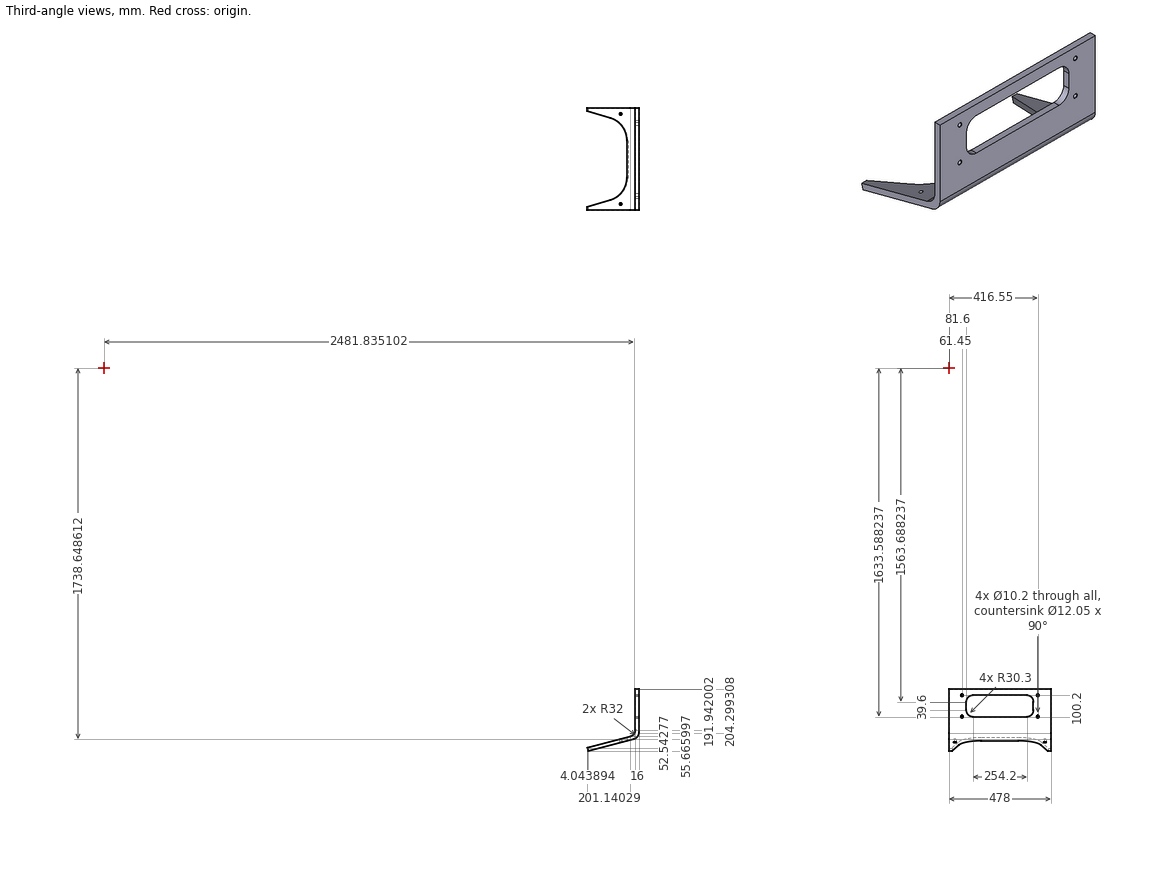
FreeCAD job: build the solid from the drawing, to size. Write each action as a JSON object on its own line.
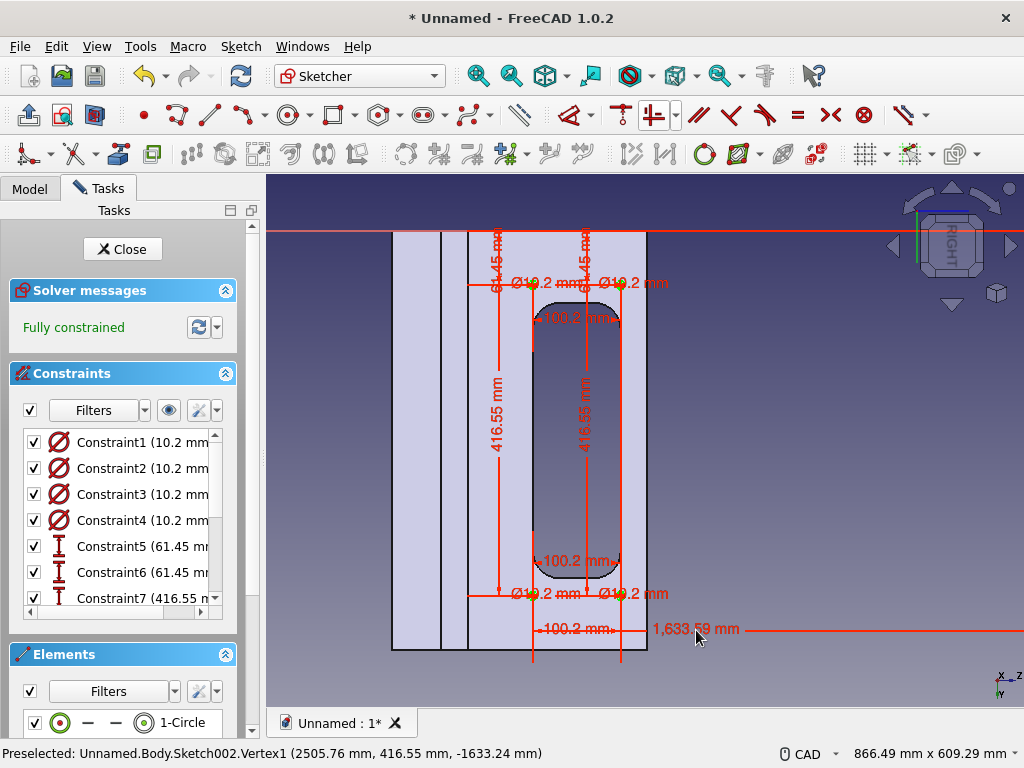
{"action": "left_click", "coordinate": [123, 249]}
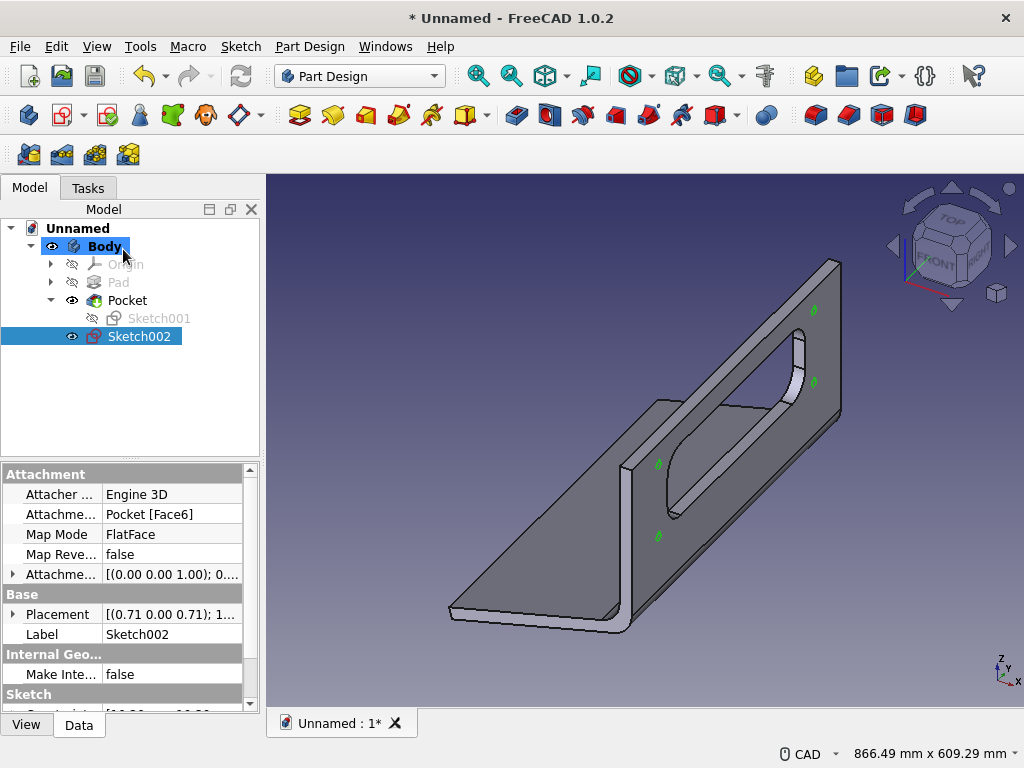
{"action": "left_click", "coordinate": [550, 116]}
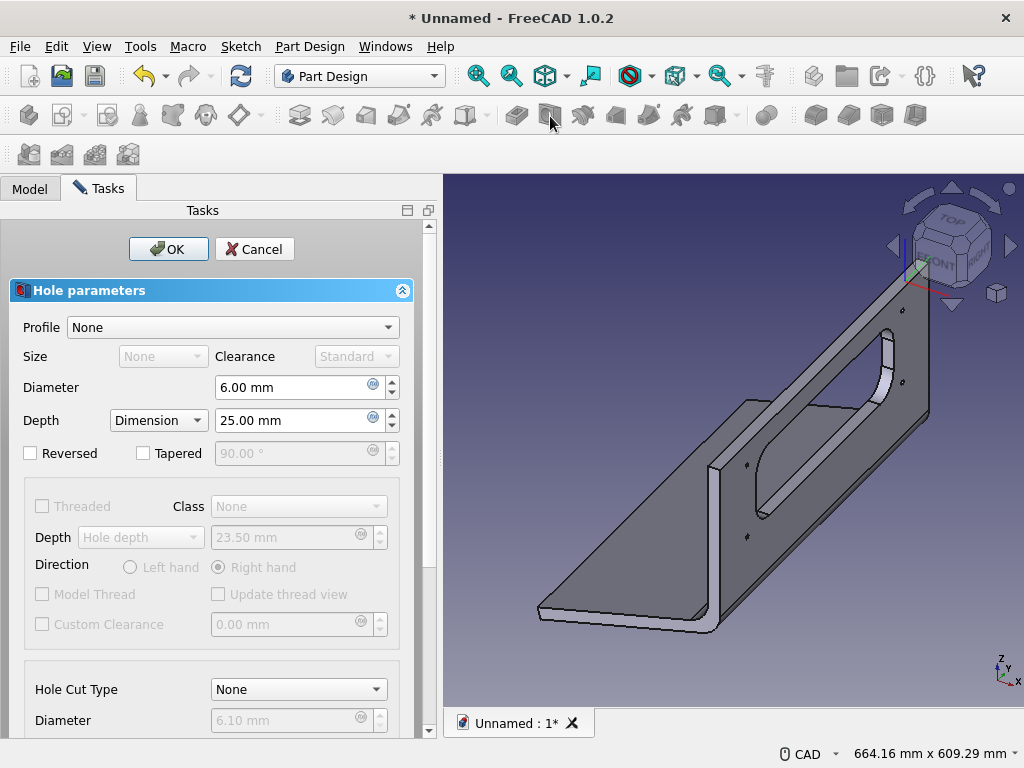
{"action": "triple_click", "coordinate": [300, 388]}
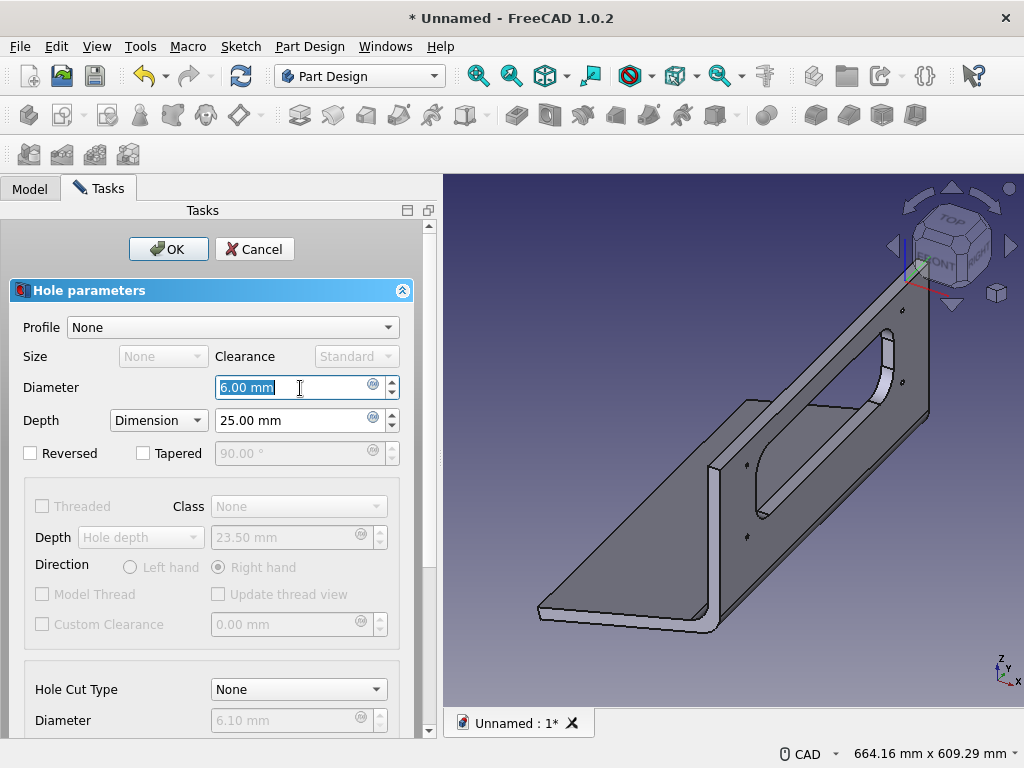
{"action": "type", "text": "10.2"}
{"action": "key", "text": "Tab"}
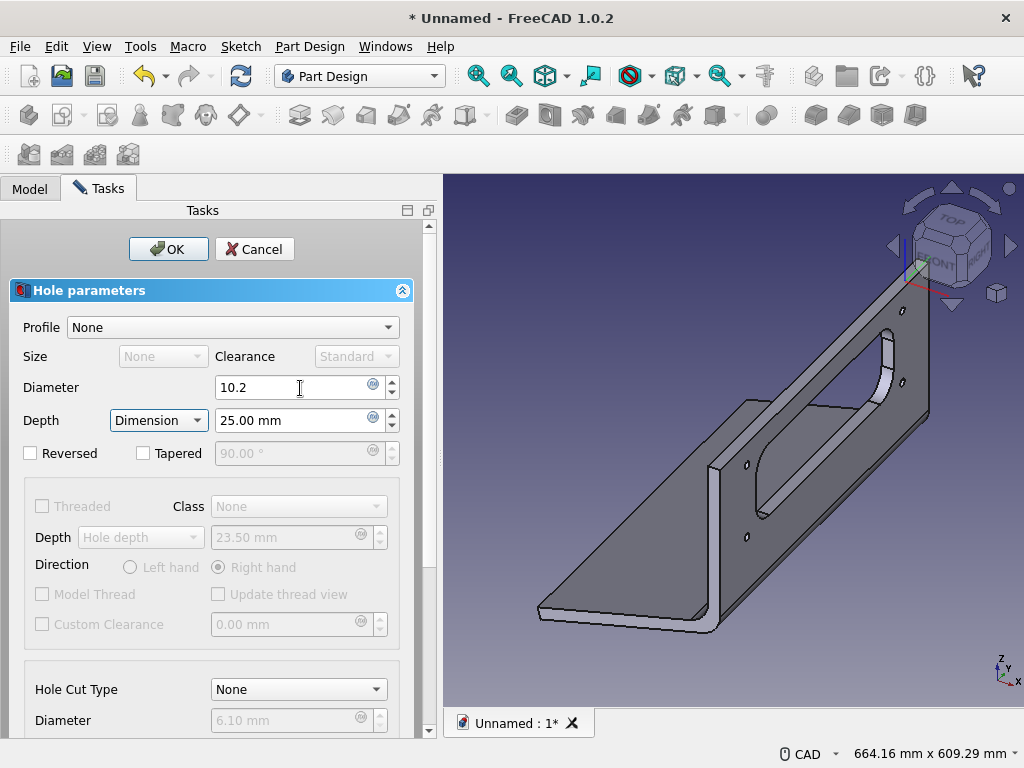
{"action": "left_click", "coordinate": [160, 420]}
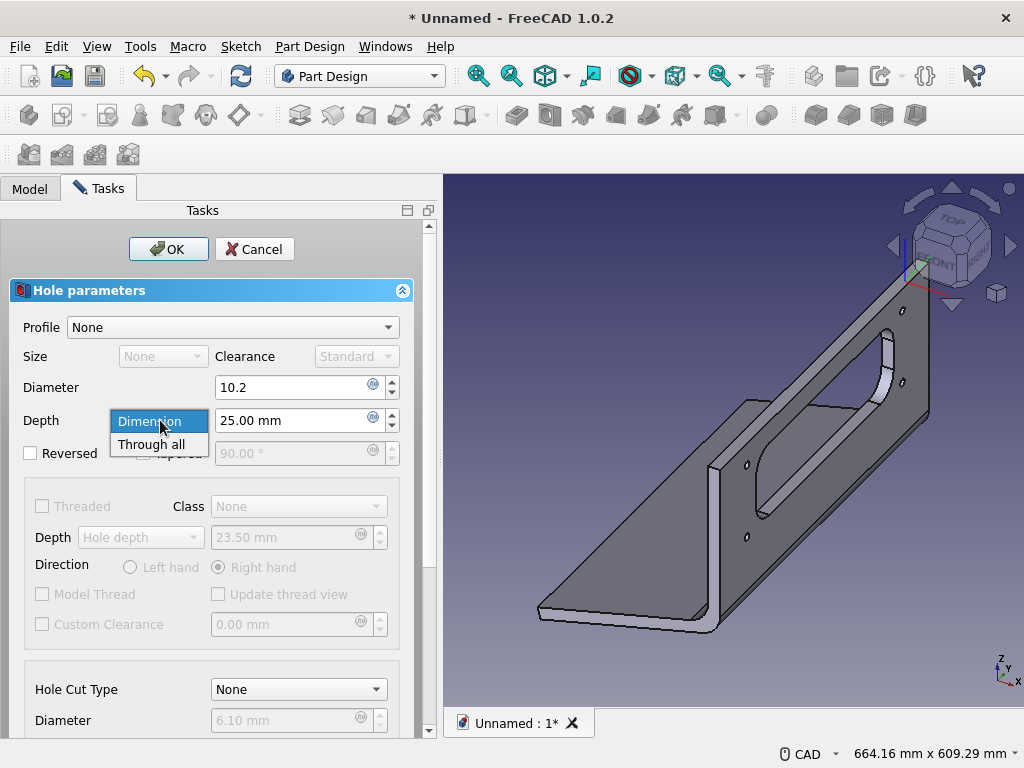
{"action": "left_click", "coordinate": [158, 444]}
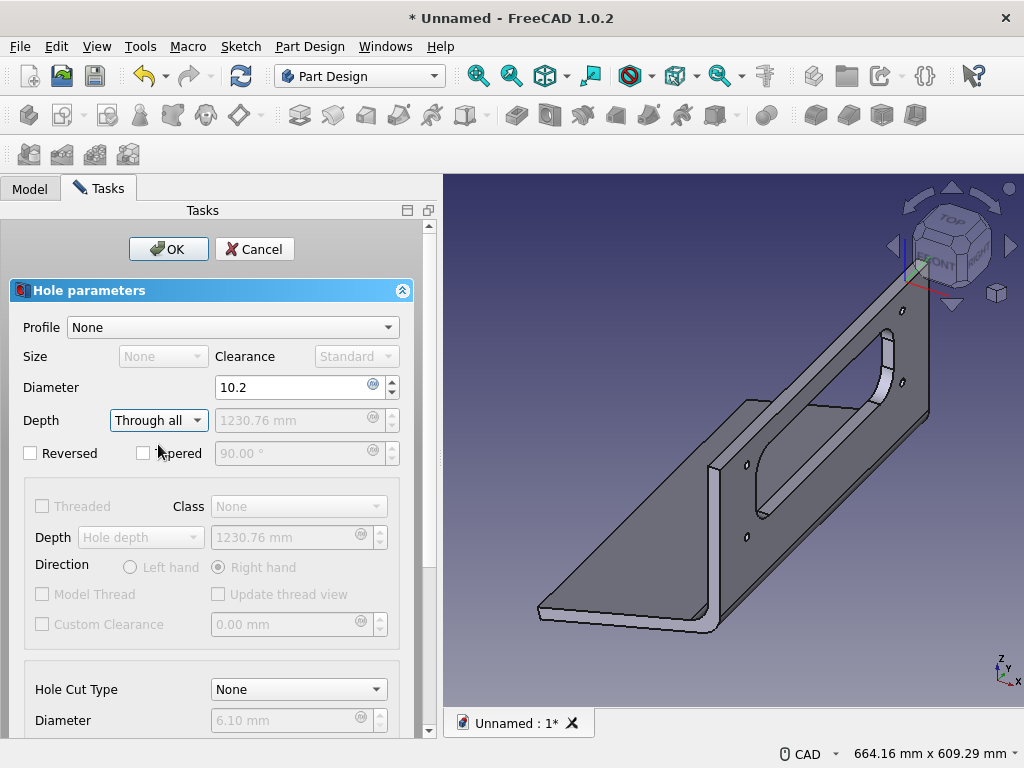
{"action": "left_click", "coordinate": [300, 690]}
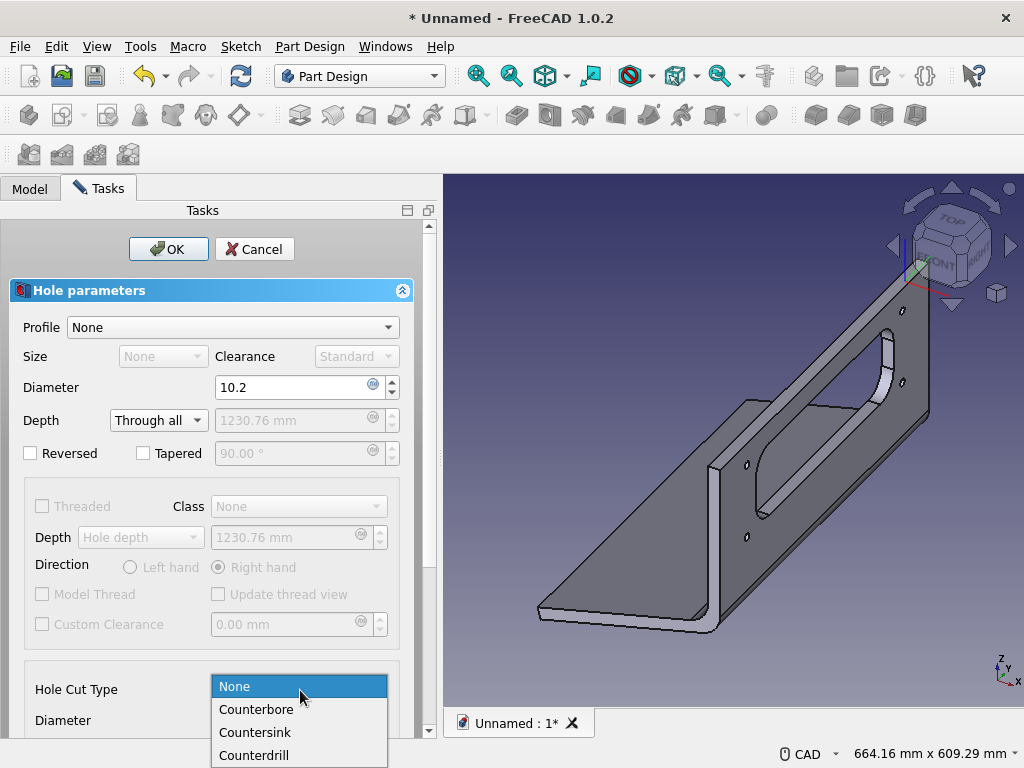
{"action": "left_click", "coordinate": [298, 732]}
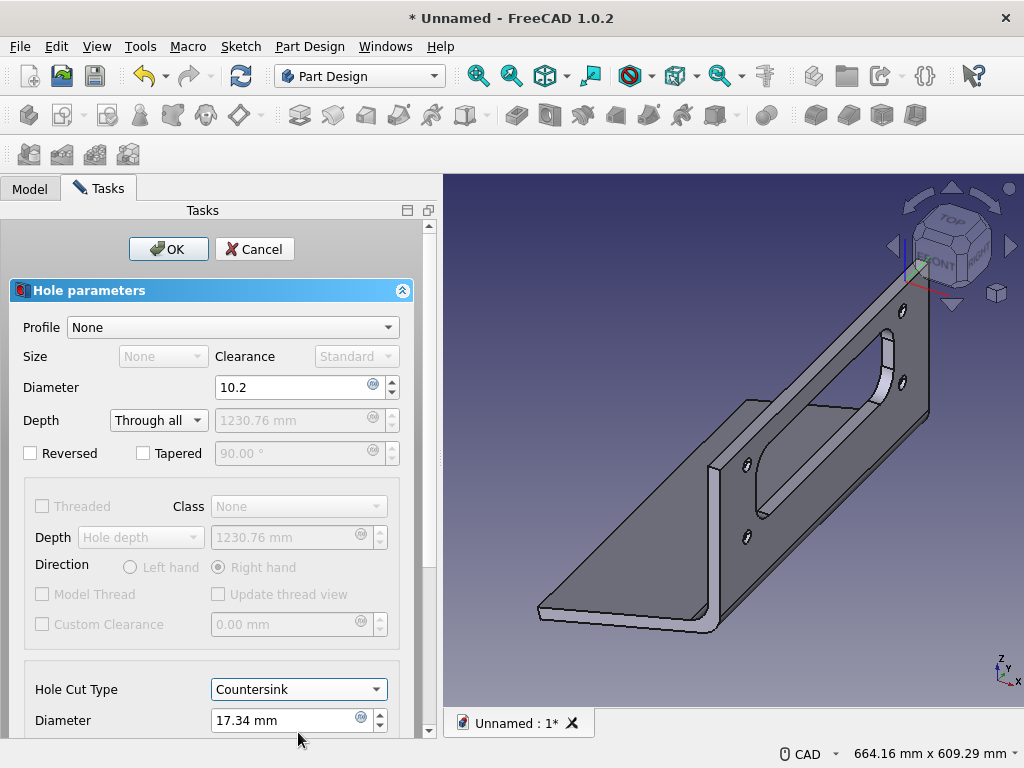
{"action": "triple_click", "coordinate": [292, 720]}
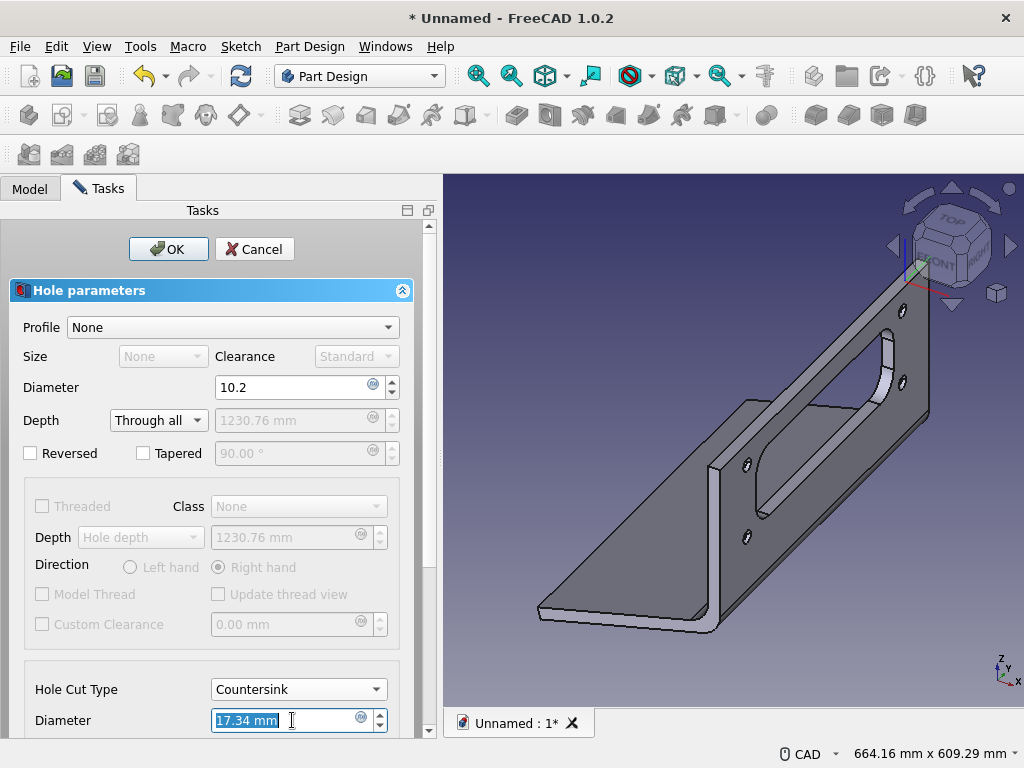
{"action": "type", "text": "12.05"}
{"action": "key", "text": "Tab"}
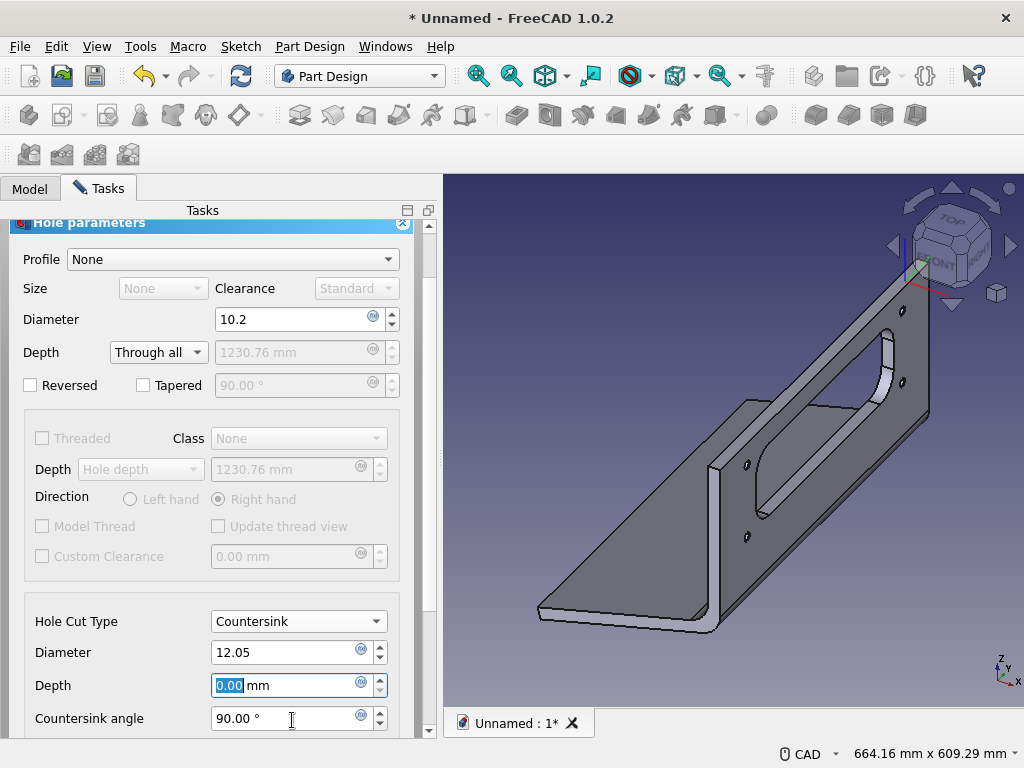
{"action": "scroll", "coordinate": [429, 479], "scroll_direction": "up", "scroll_amount": 2}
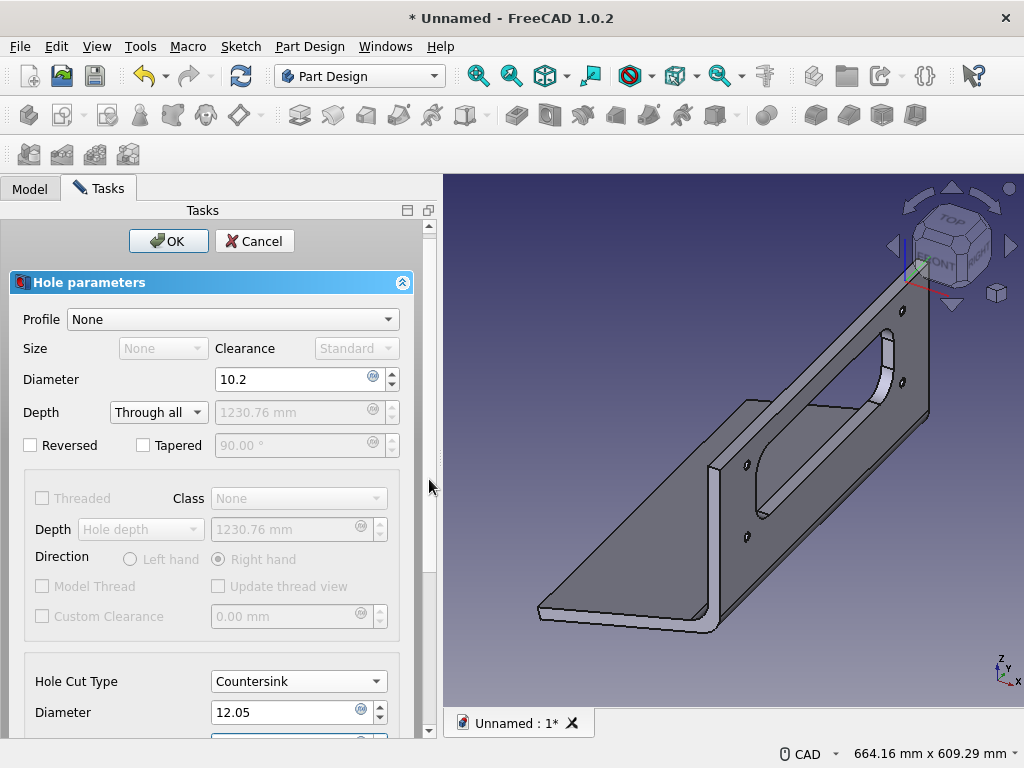
{"action": "left_click", "coordinate": [169, 249]}